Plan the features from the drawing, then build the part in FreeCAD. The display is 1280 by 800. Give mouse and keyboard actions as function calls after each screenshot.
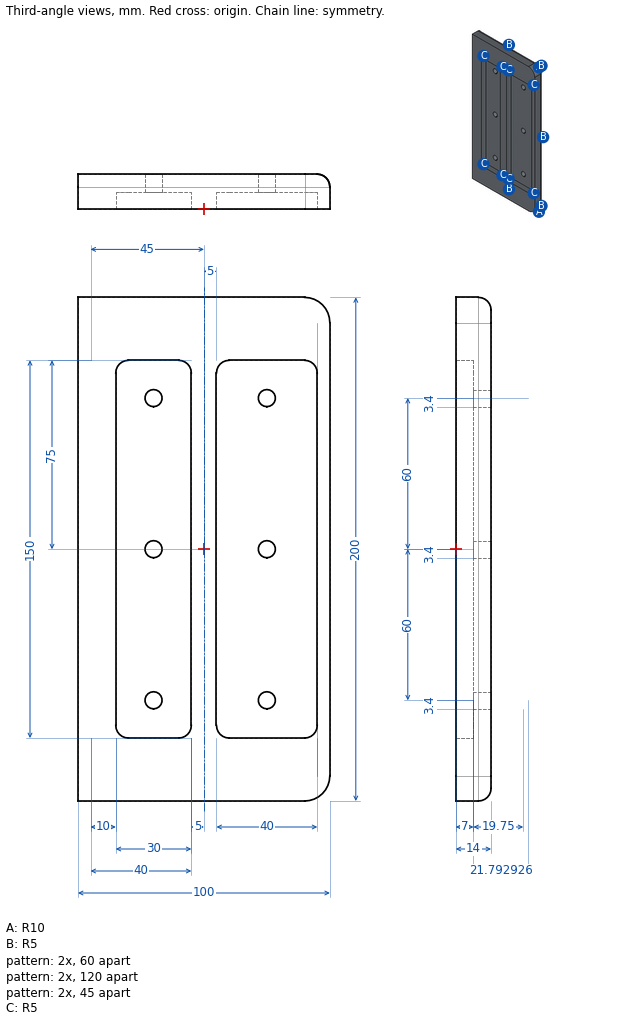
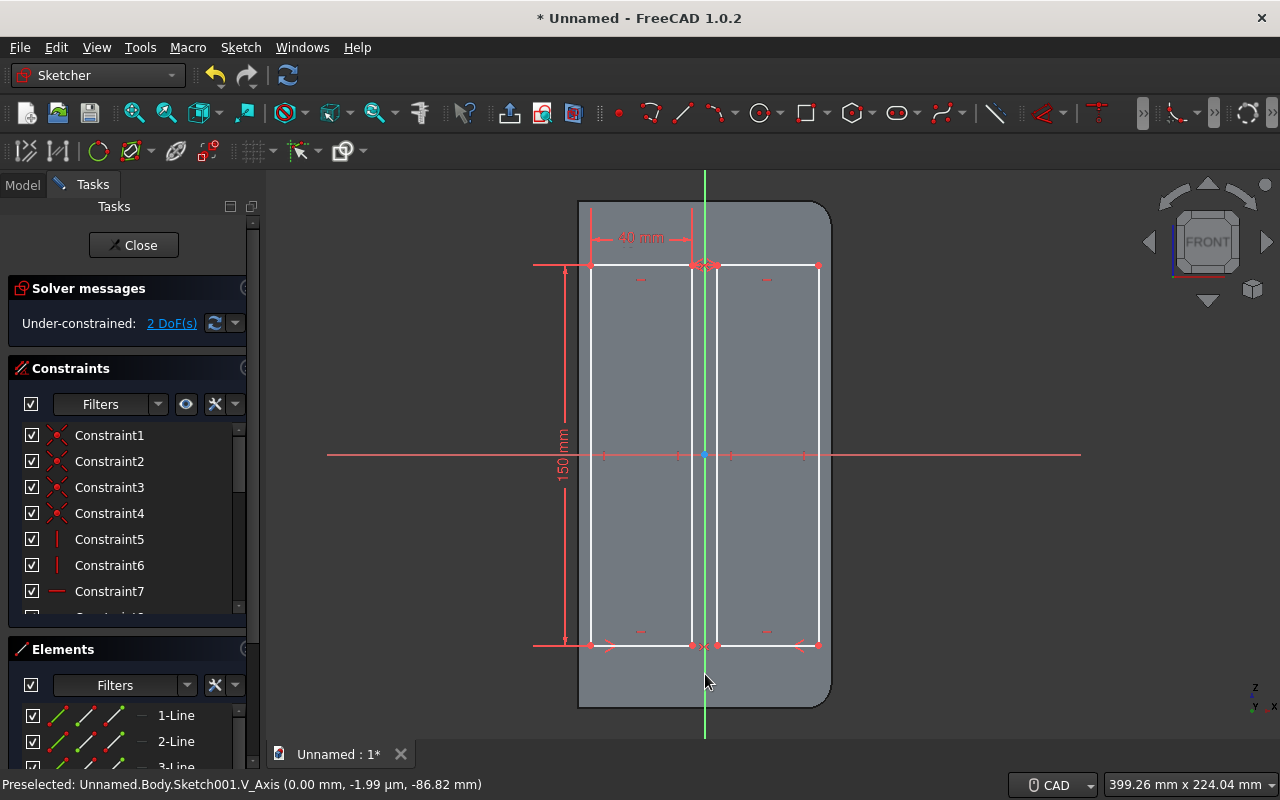
click(1042, 114)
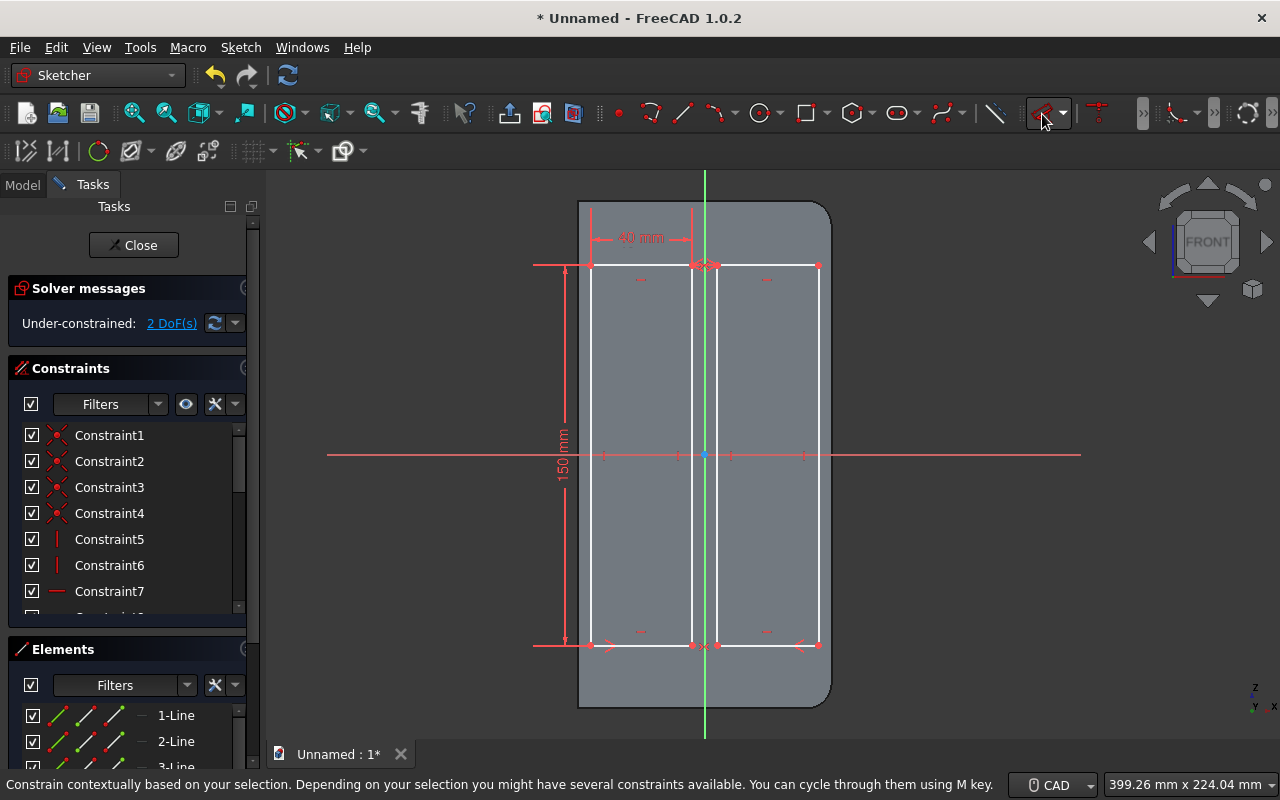
scroll(692, 646, up, 6)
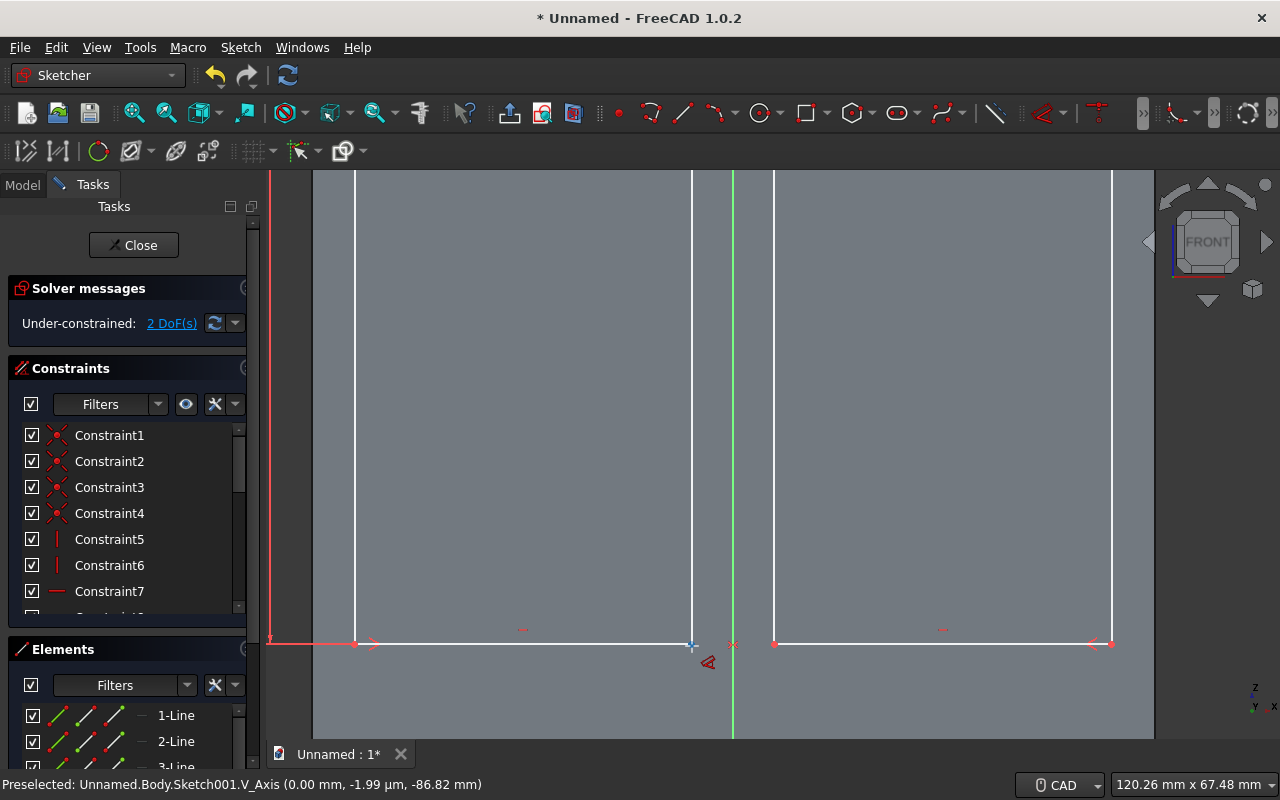
click(692, 644)
click(713, 678)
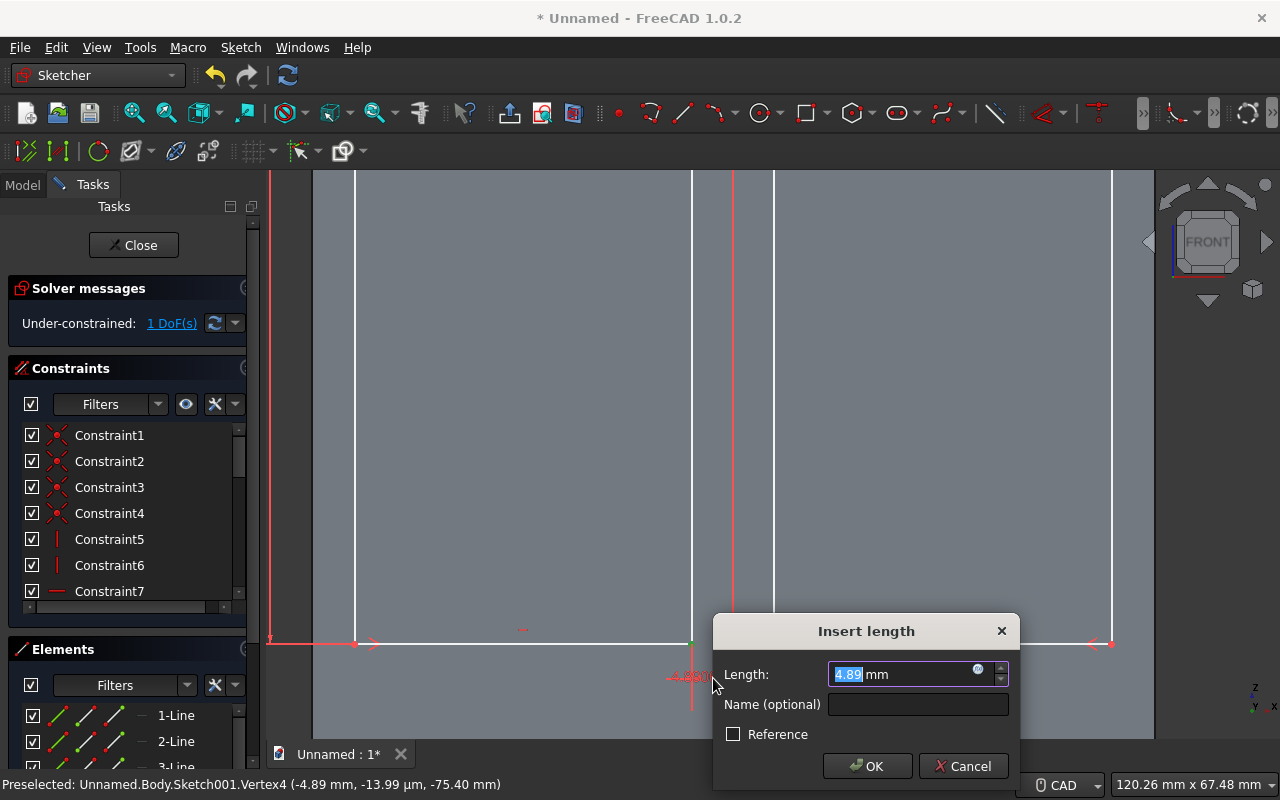
text(5)
key(Return)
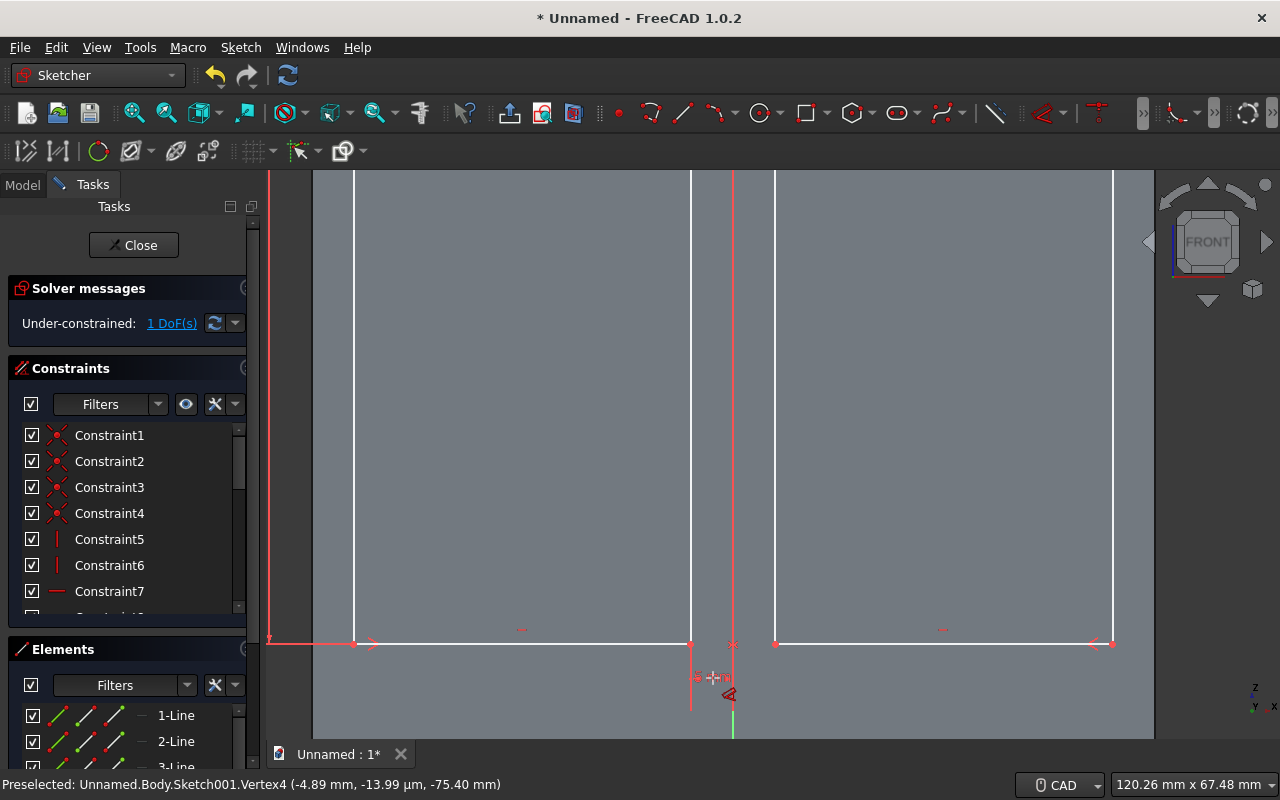
scroll(692, 647, down, 6)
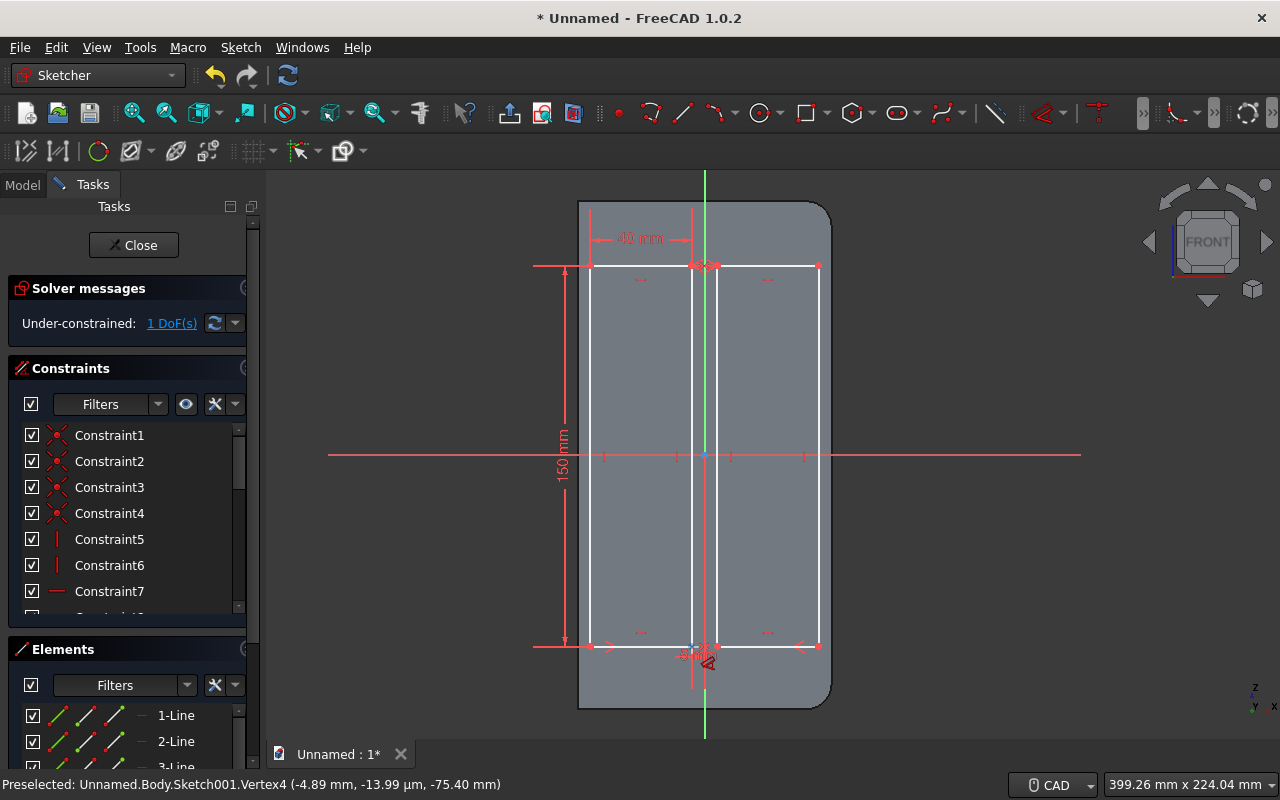
click(590, 266)
click(556, 360)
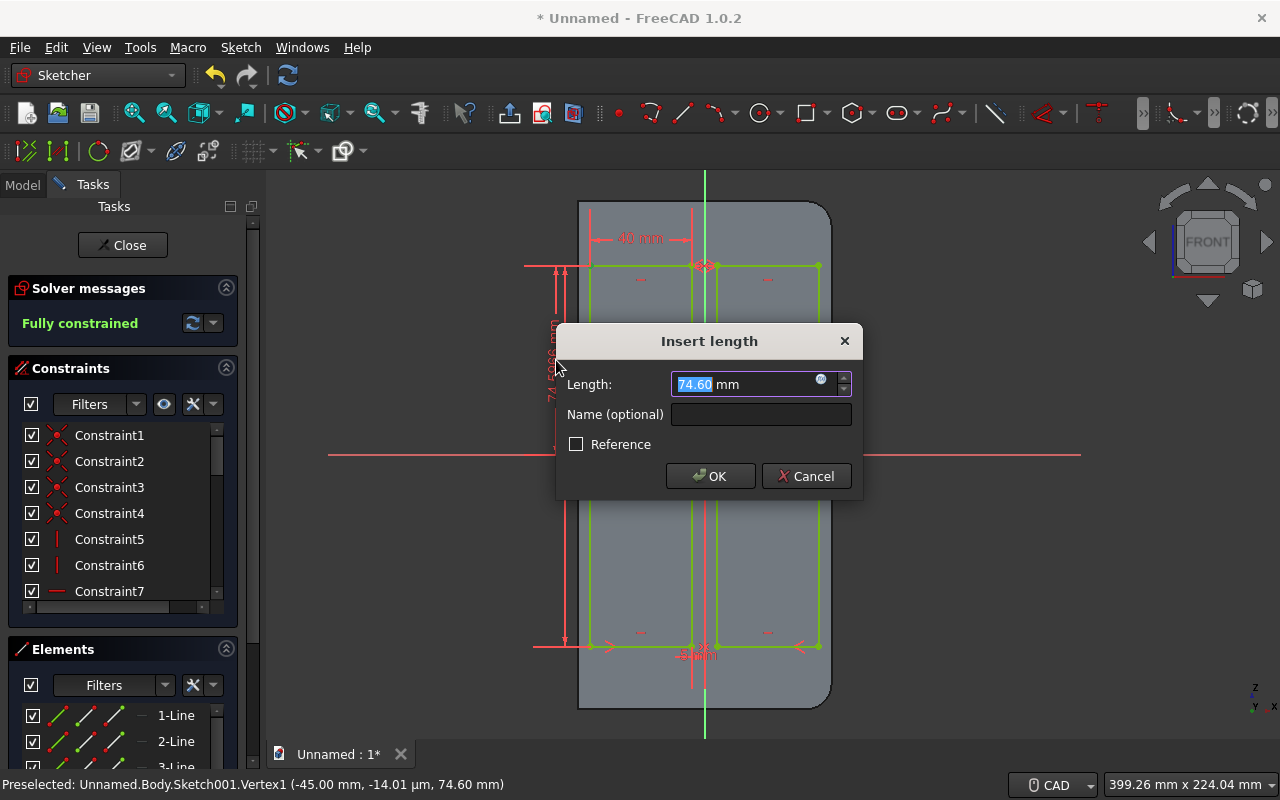
text(75)
key(Return)
key(Escape)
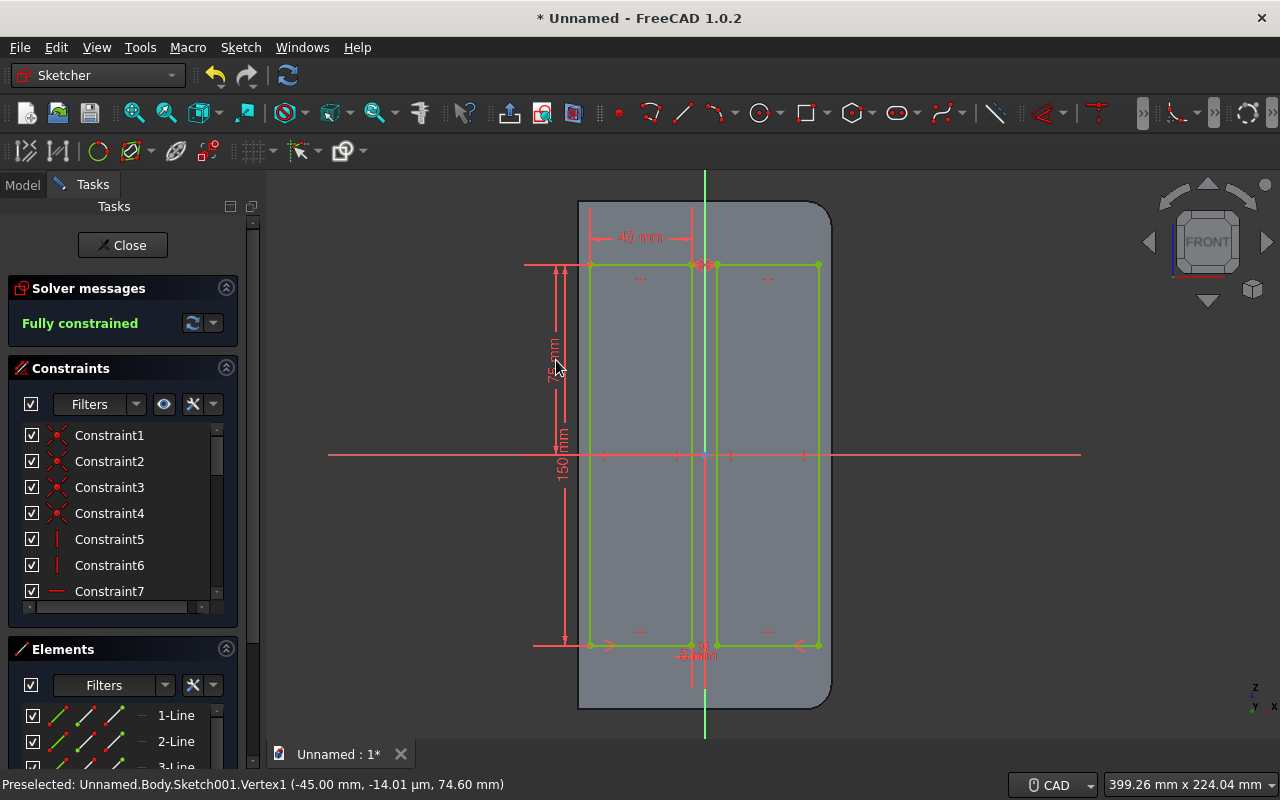
click(123, 245)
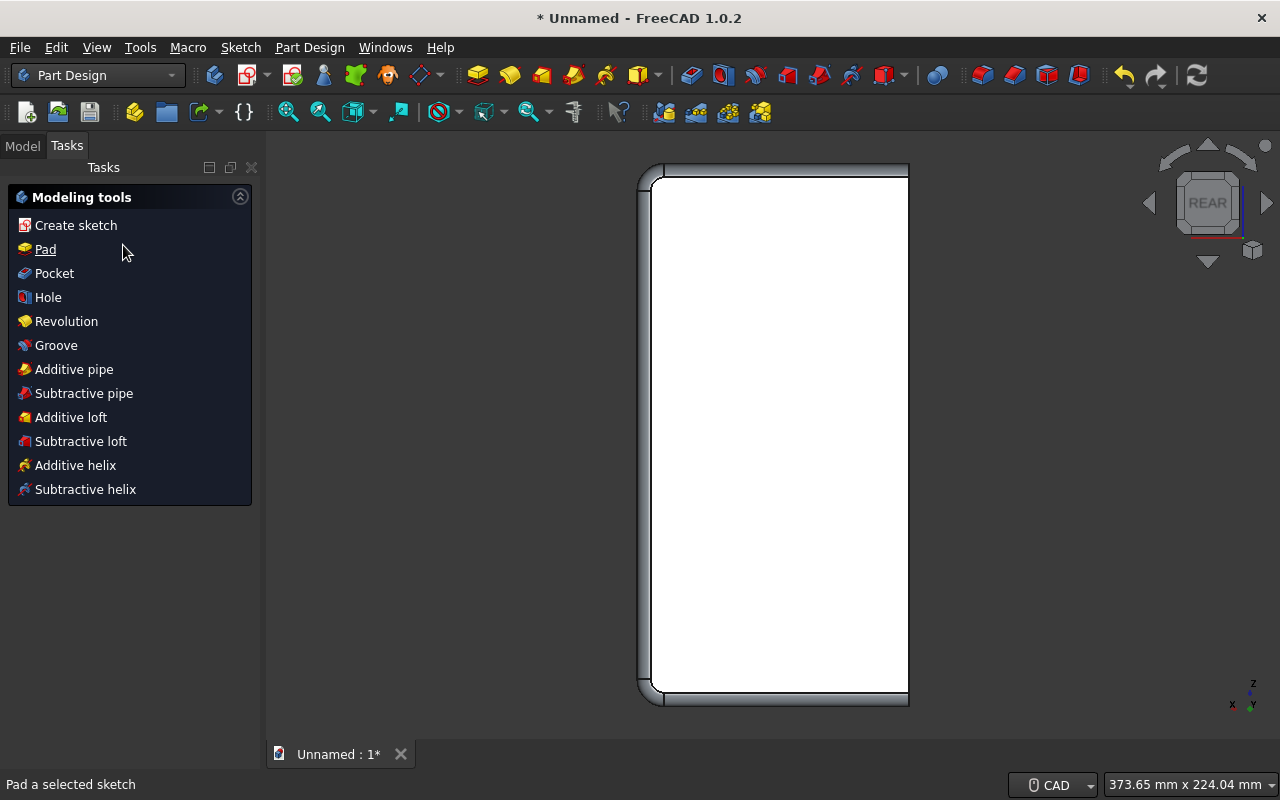
click(478, 76)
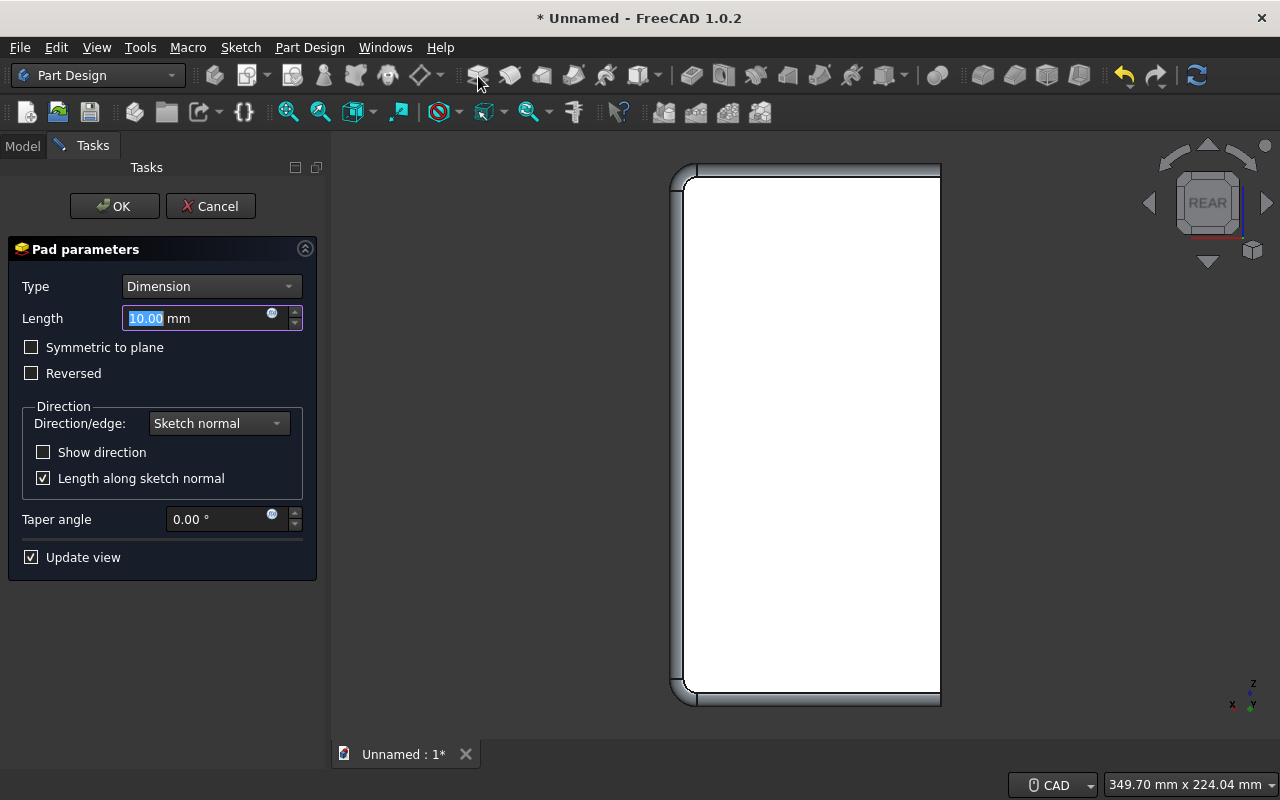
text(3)
key(Tab)